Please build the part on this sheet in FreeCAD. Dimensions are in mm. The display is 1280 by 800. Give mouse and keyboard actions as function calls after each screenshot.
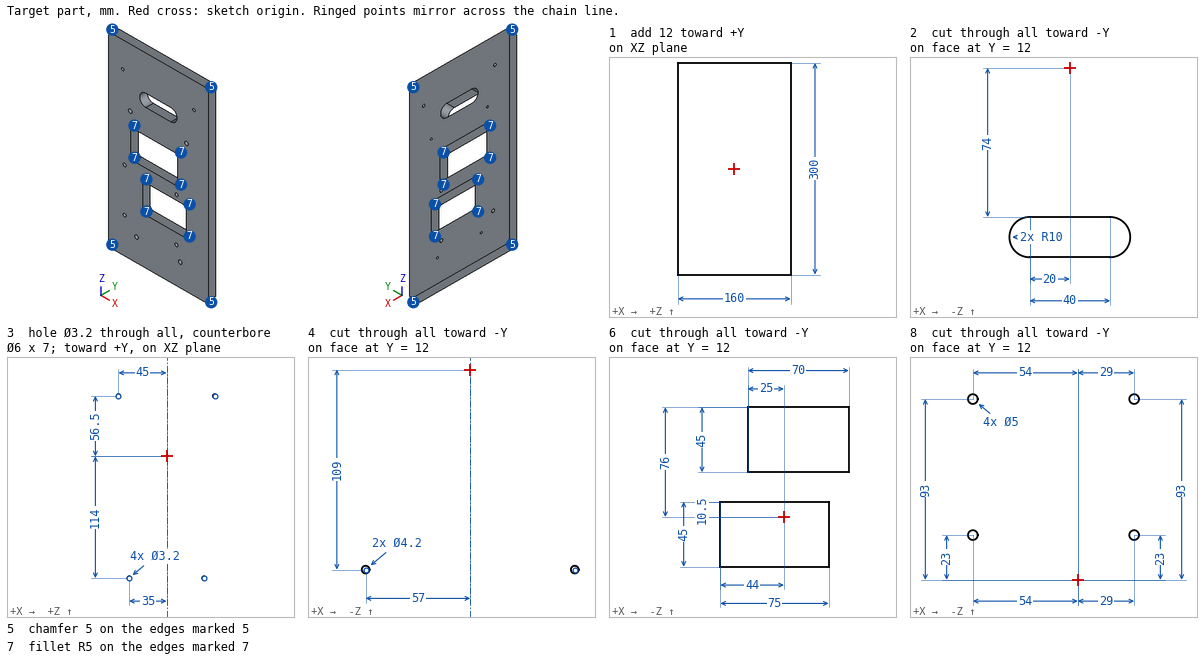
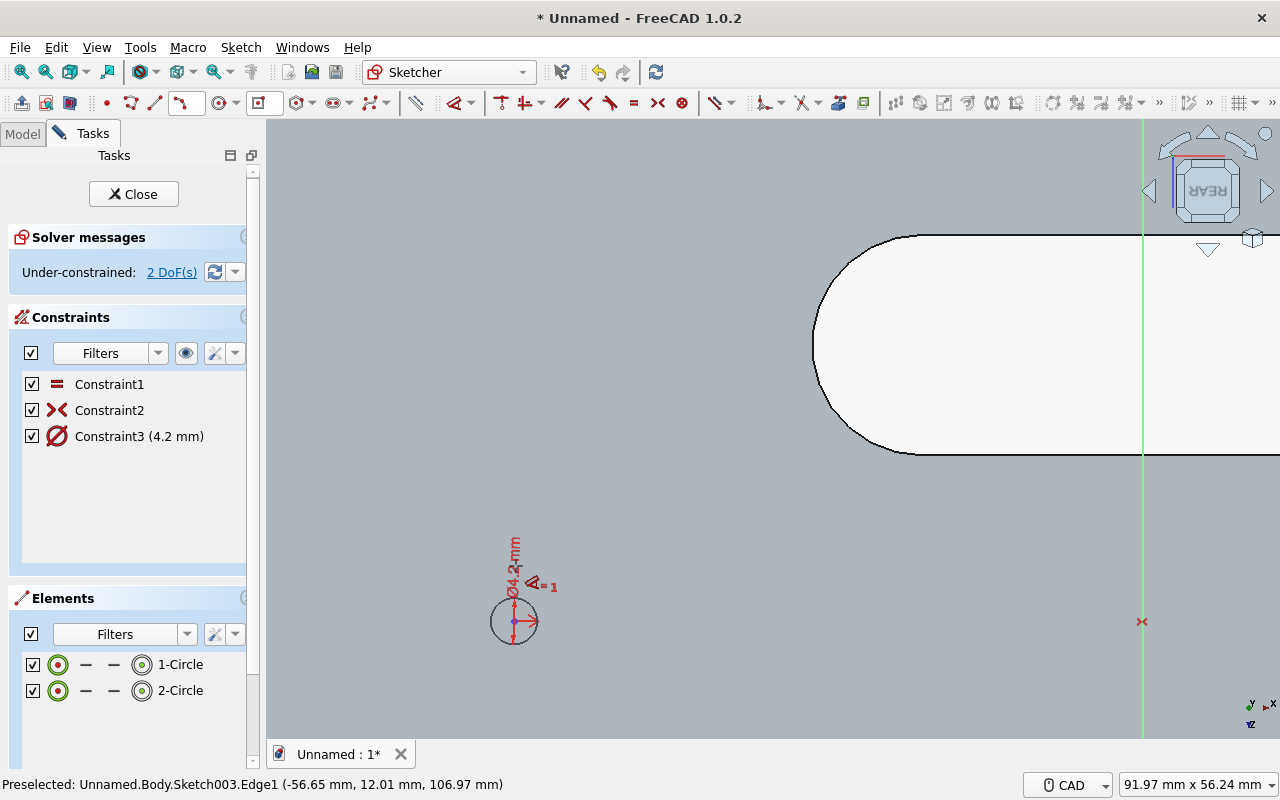
click(514, 621)
click(815, 655)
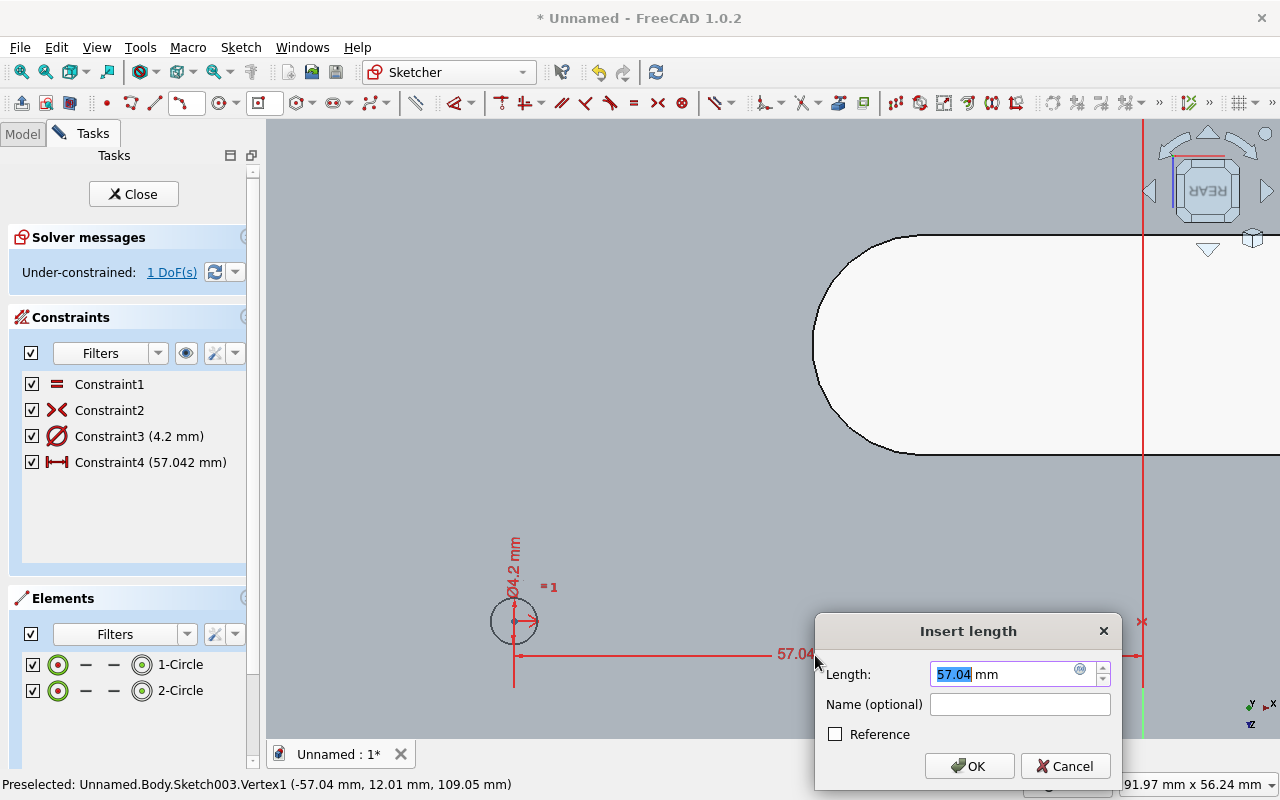
text(57)
key(Return)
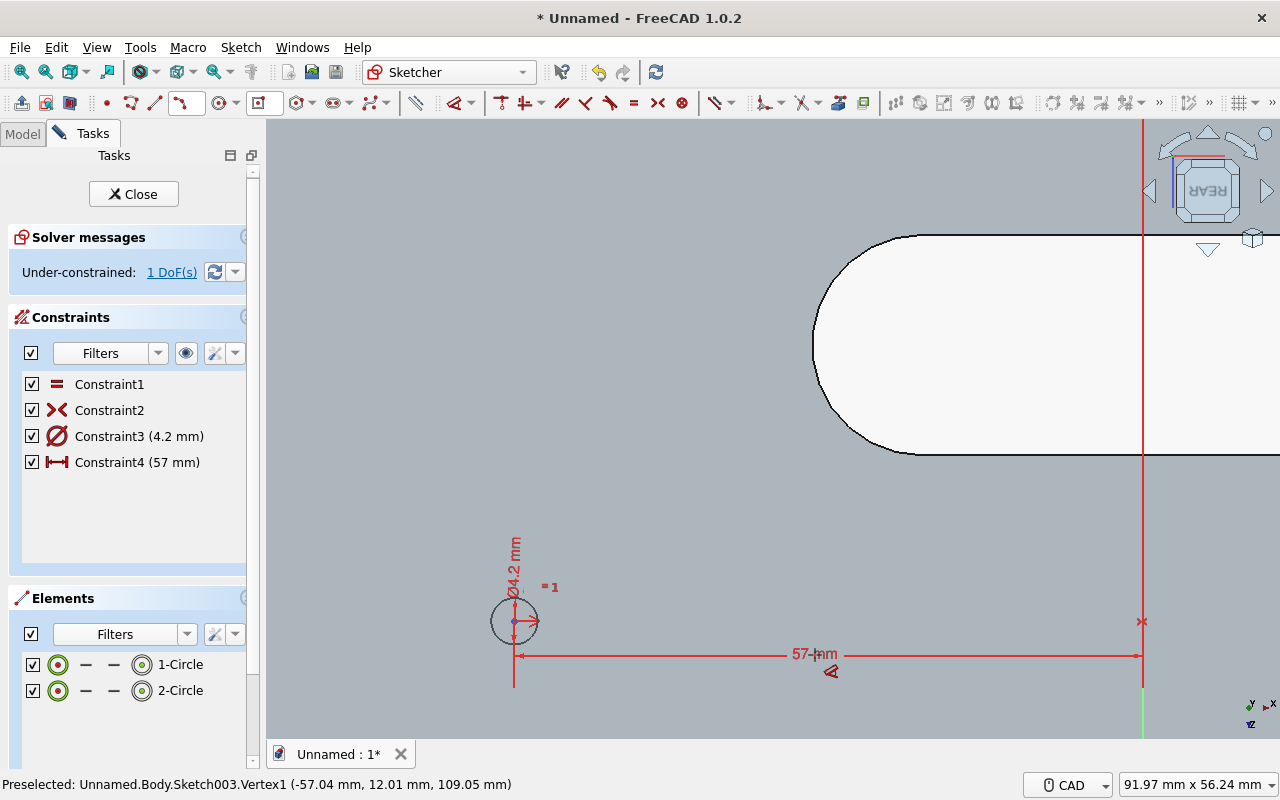
click(514, 621)
click(480, 384)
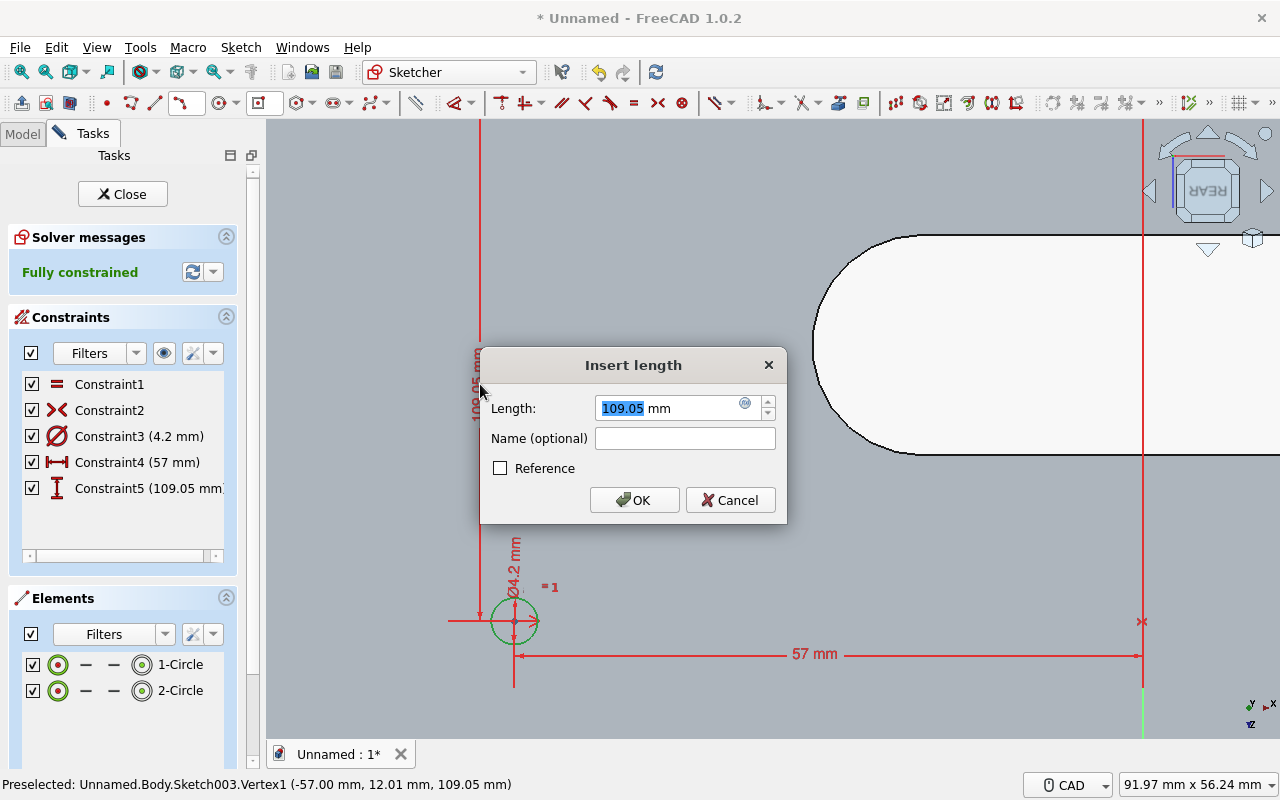
text(109)
key(Return)
key(Escape)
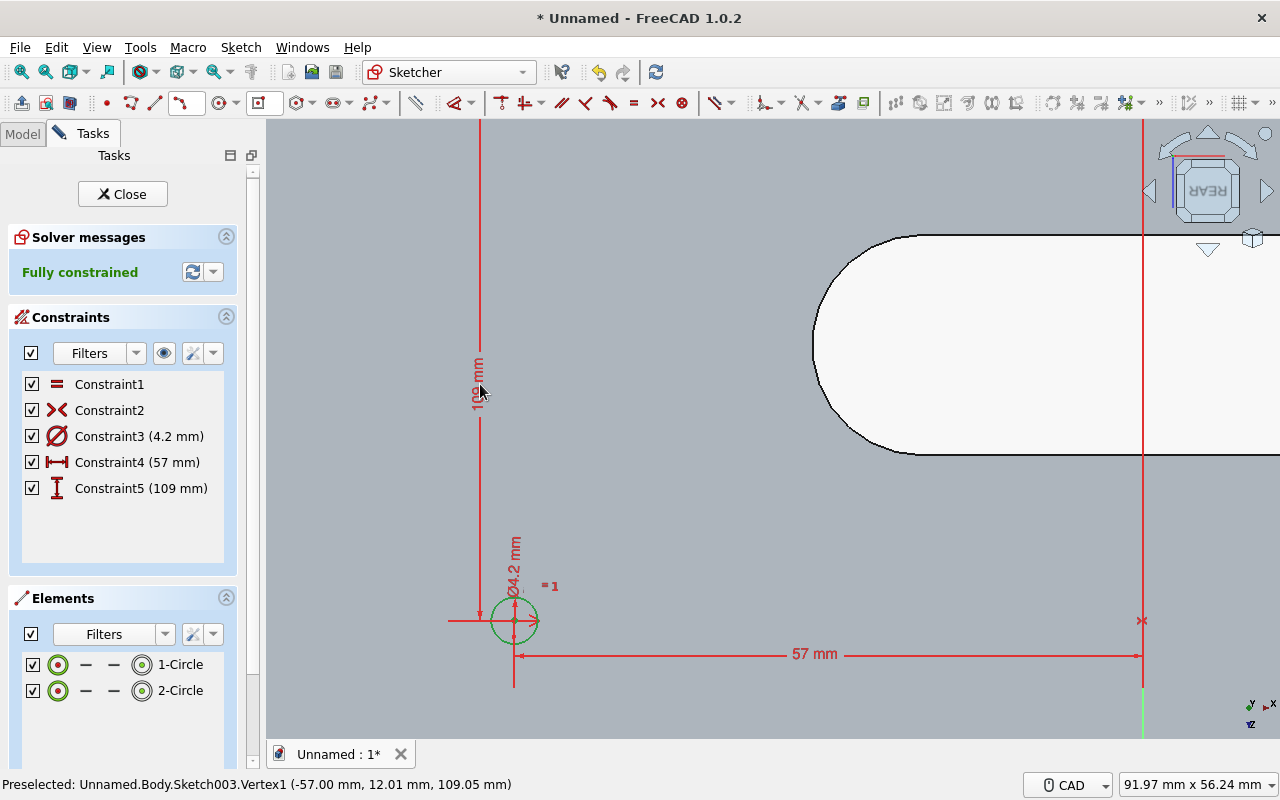
click(123, 194)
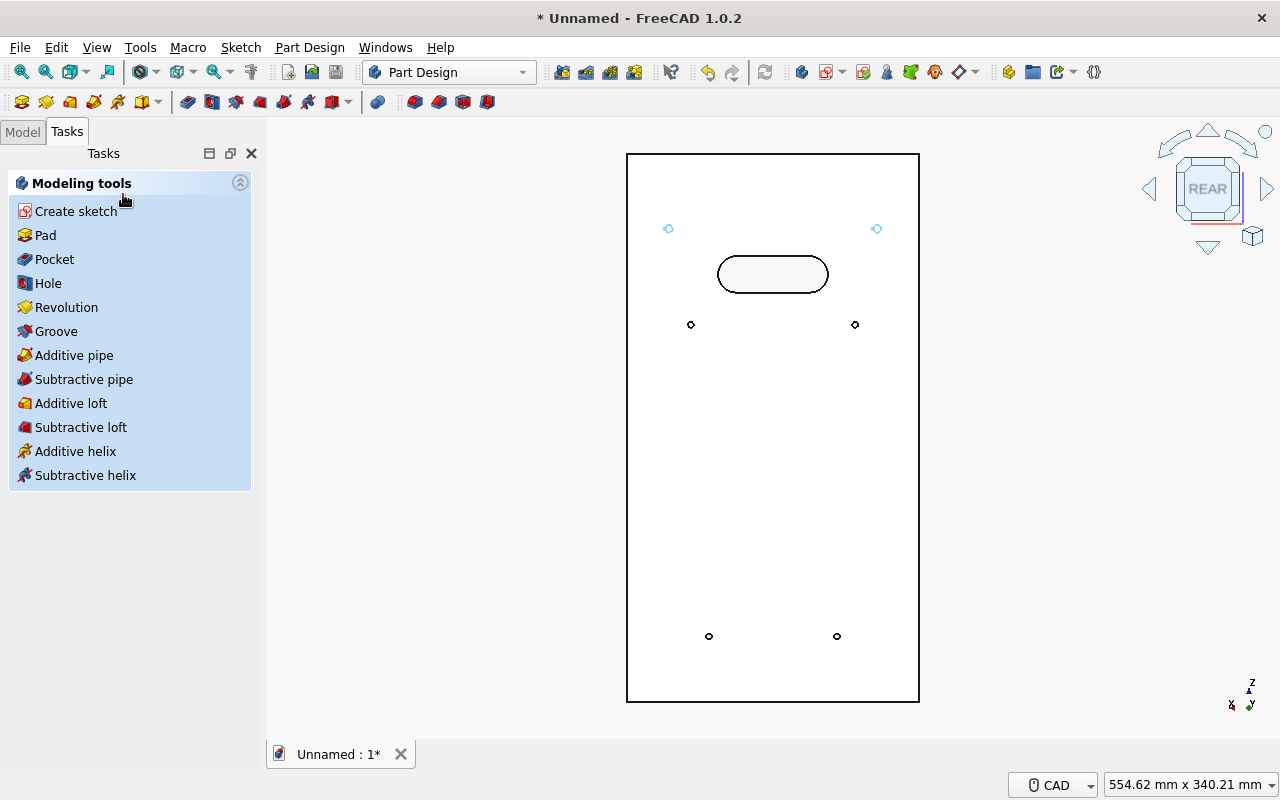
click(188, 102)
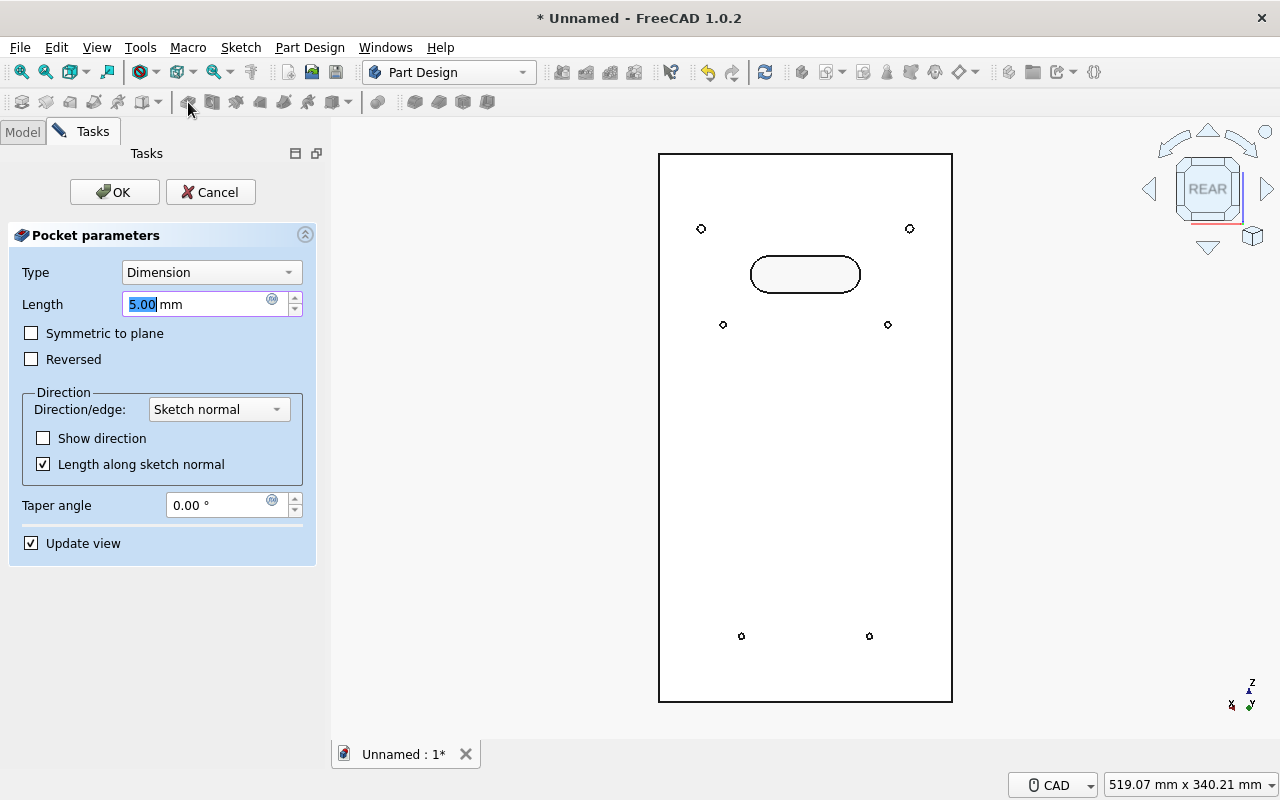
click(212, 272)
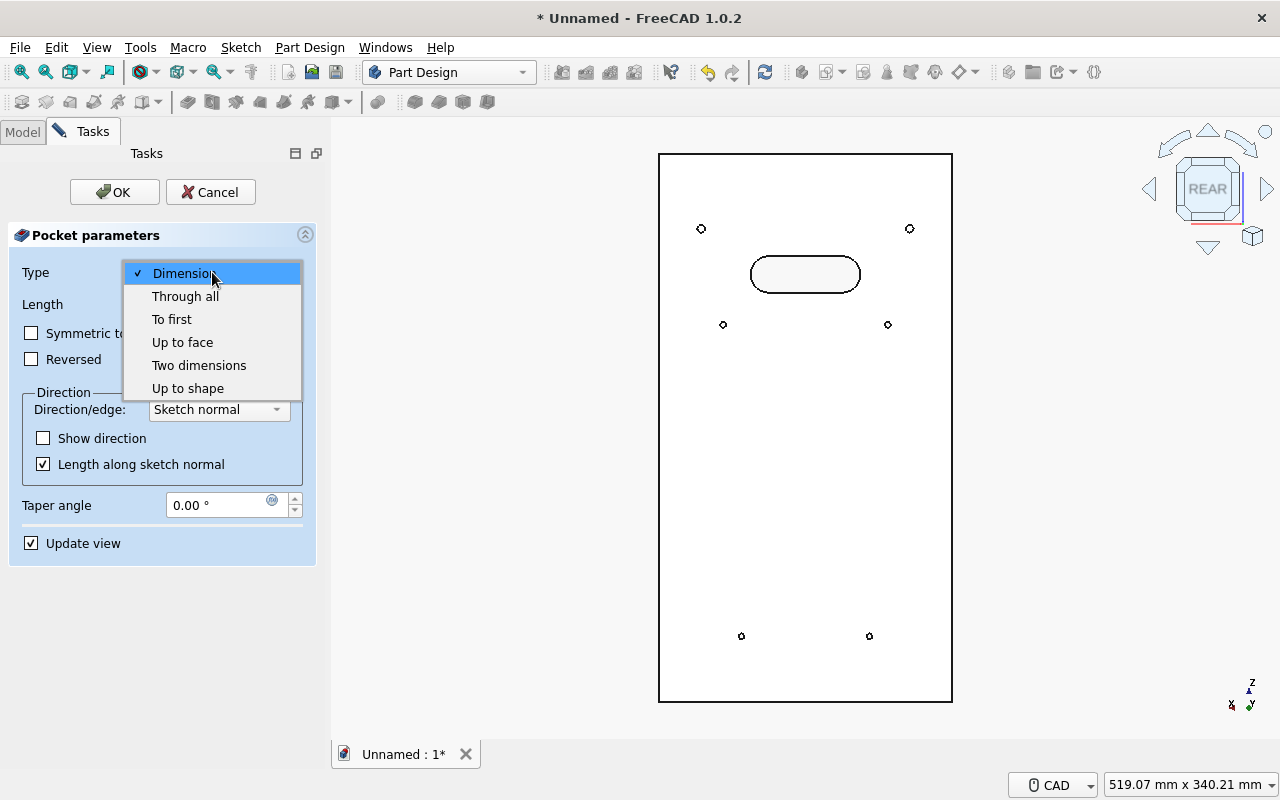
click(212, 296)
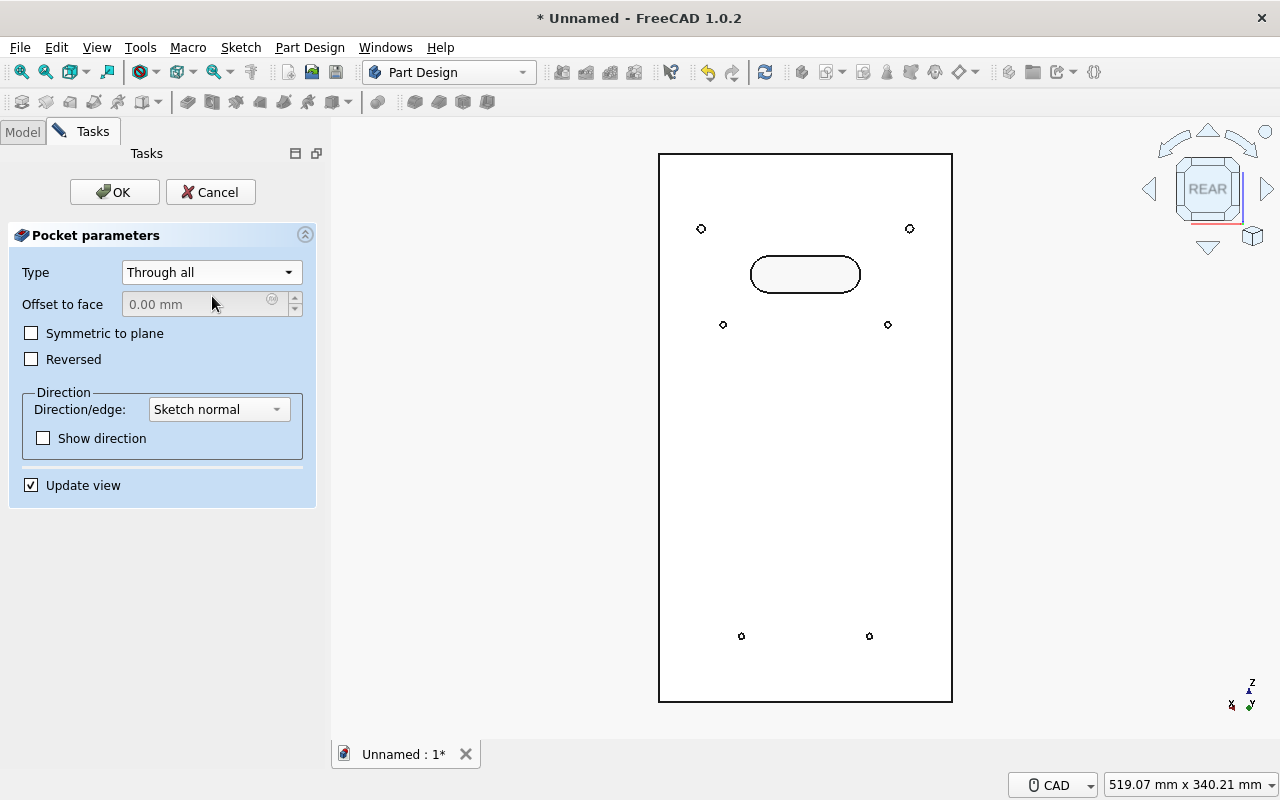
click(115, 192)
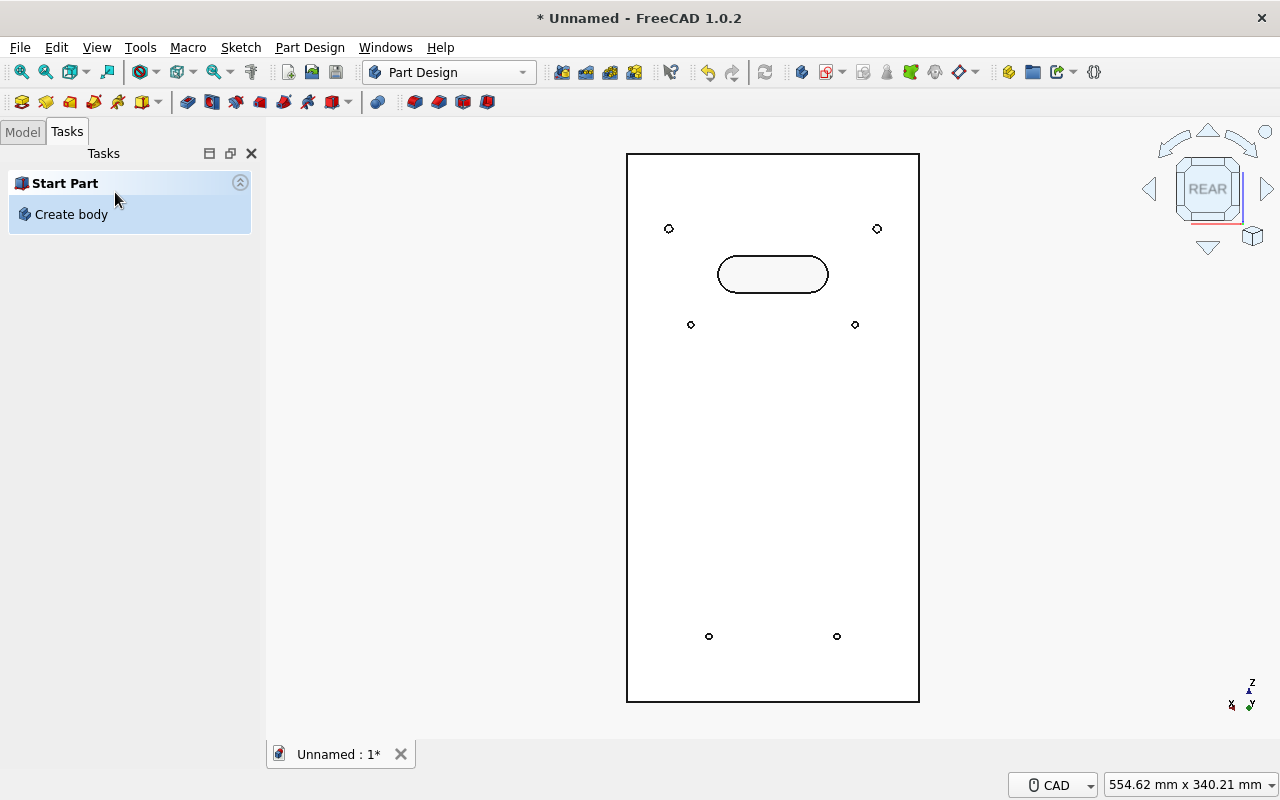
scroll(627, 153, up, 4)